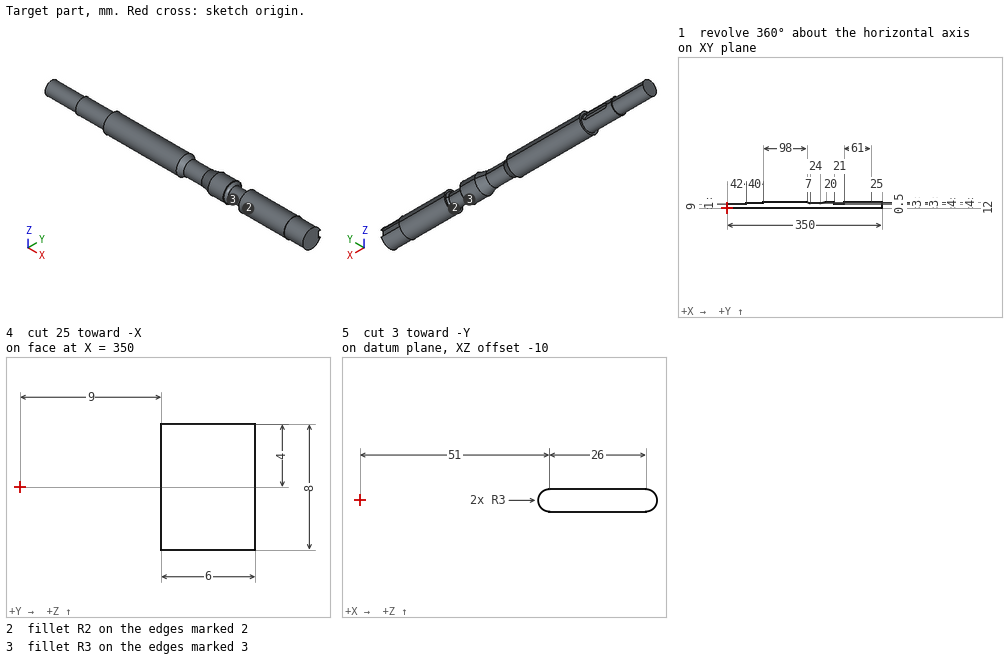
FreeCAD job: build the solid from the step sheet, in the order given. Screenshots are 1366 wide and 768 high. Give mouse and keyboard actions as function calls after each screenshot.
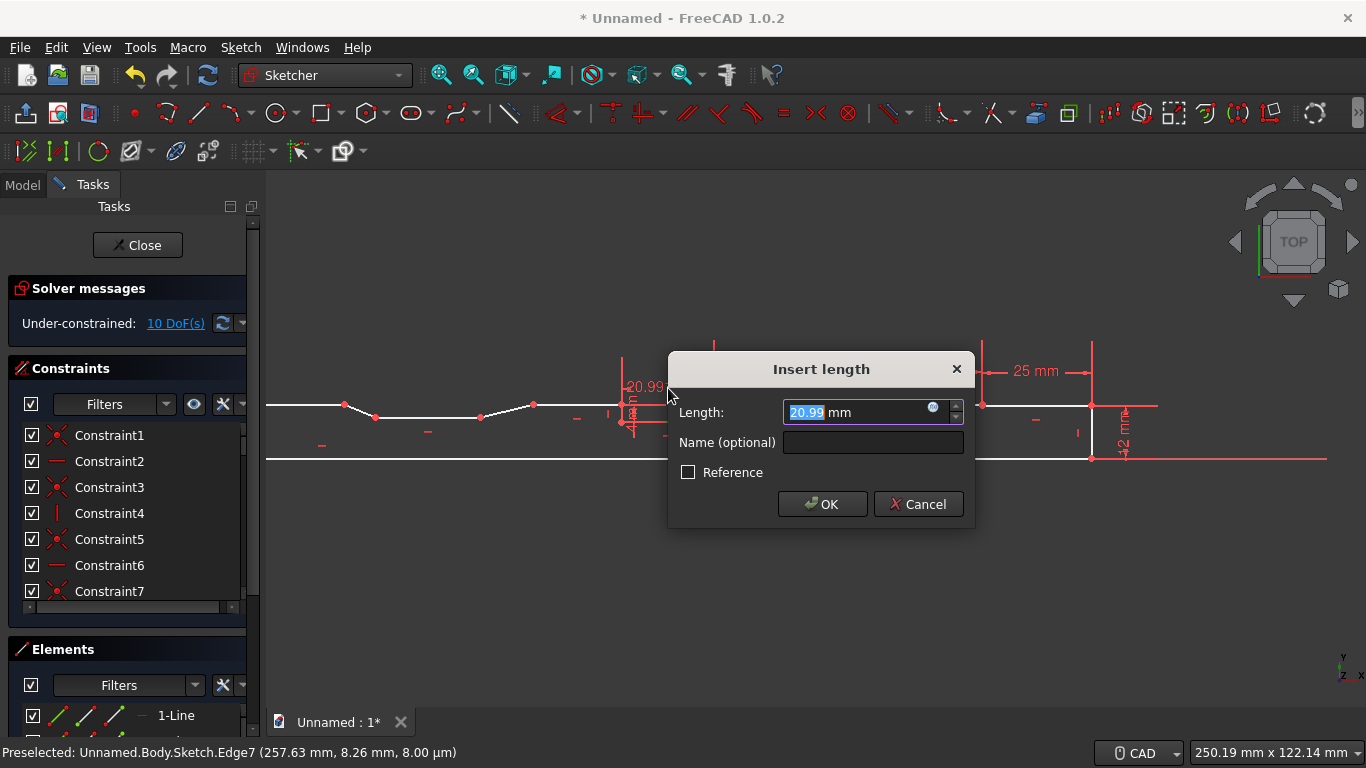
text(21)
key(Return)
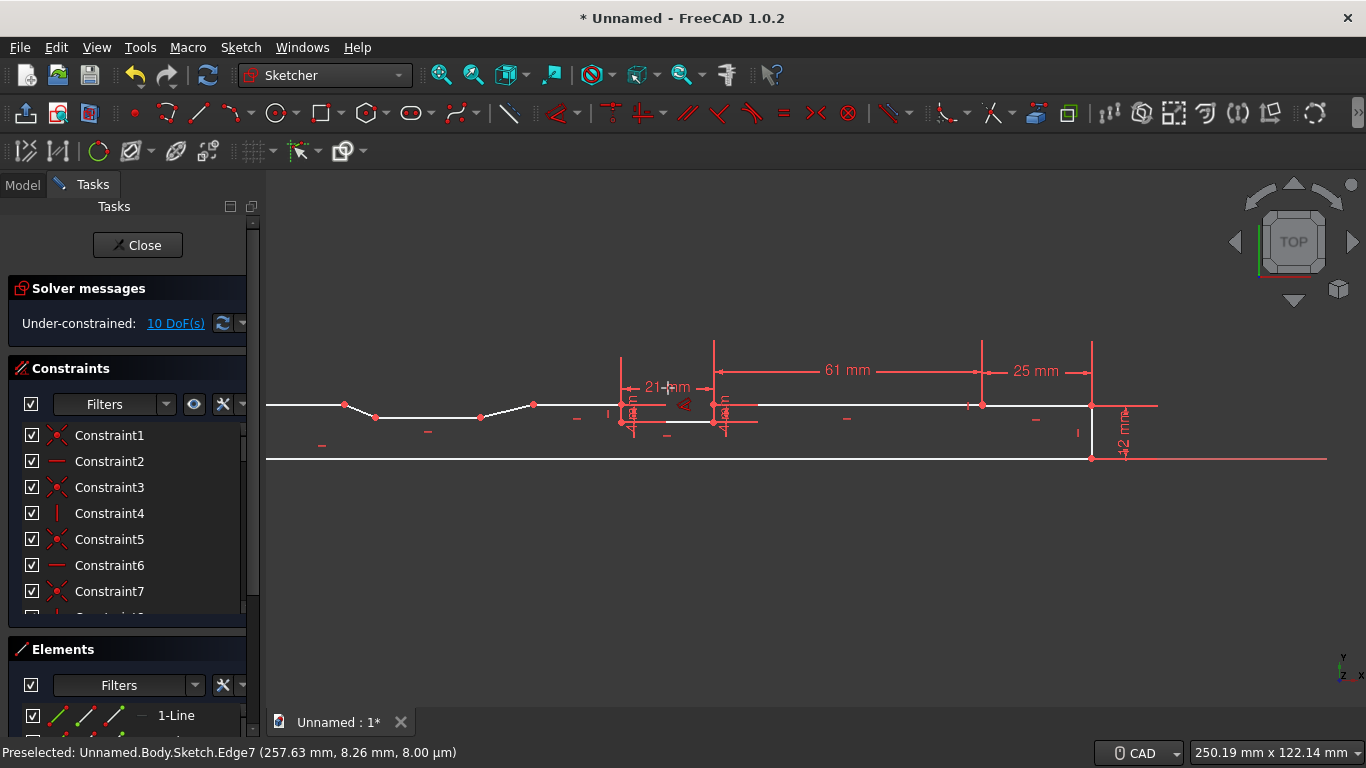
click(595, 405)
click(578, 371)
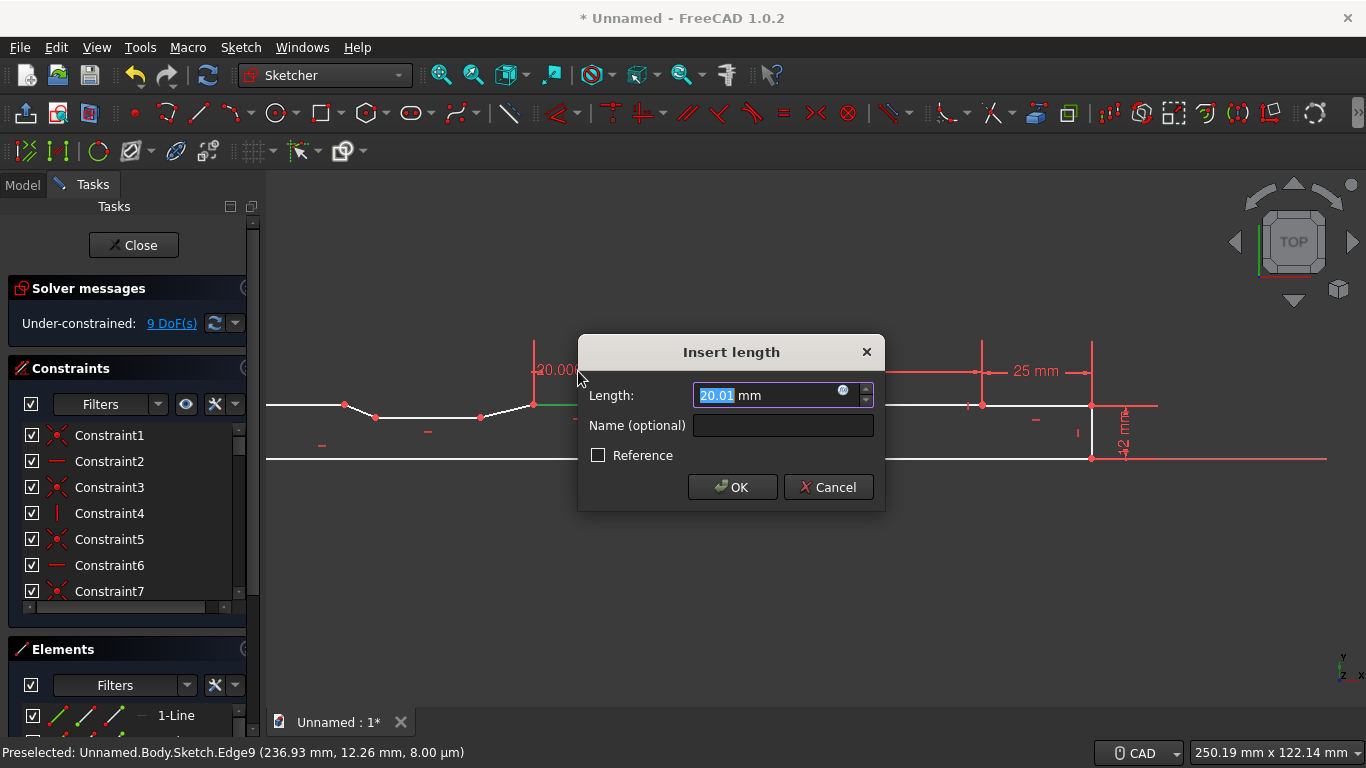
text(20)
key(Return)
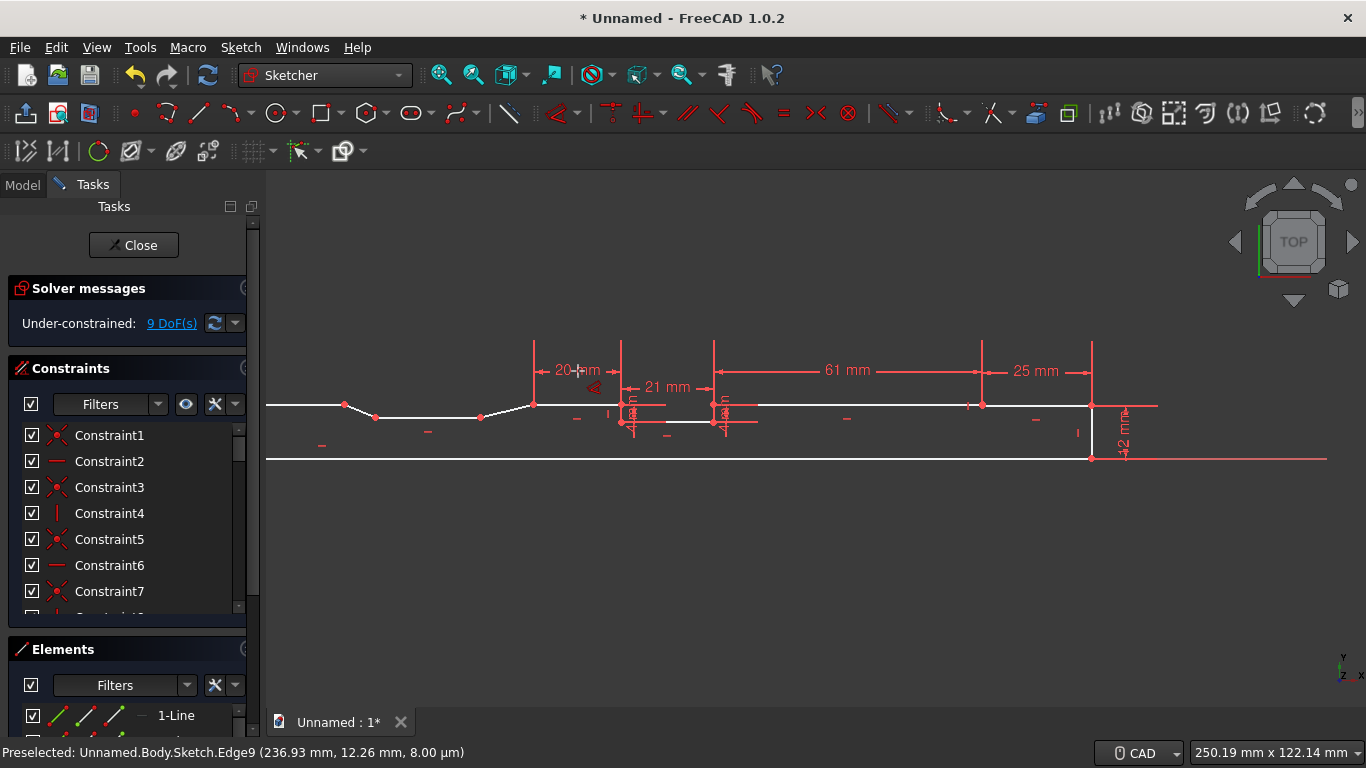
click(449, 418)
click(428, 384)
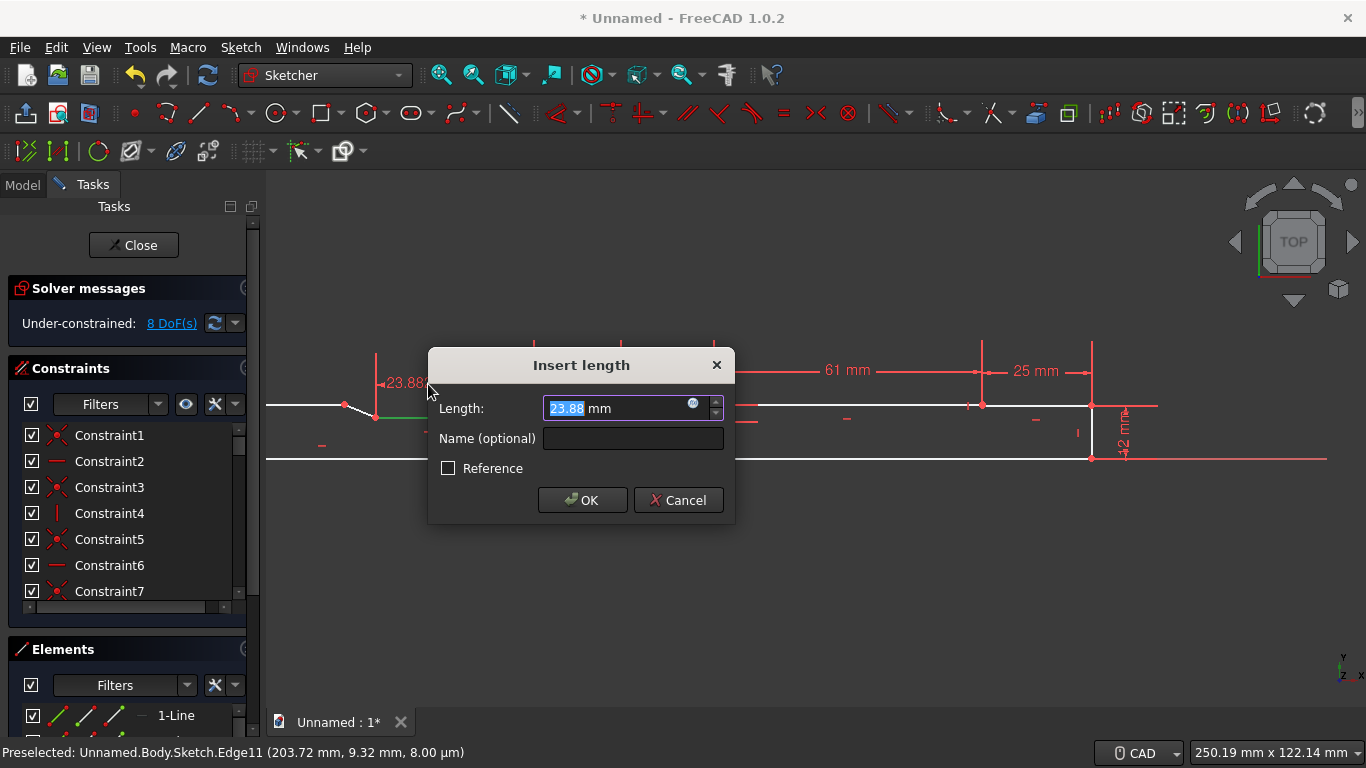
text(24)
key(Return)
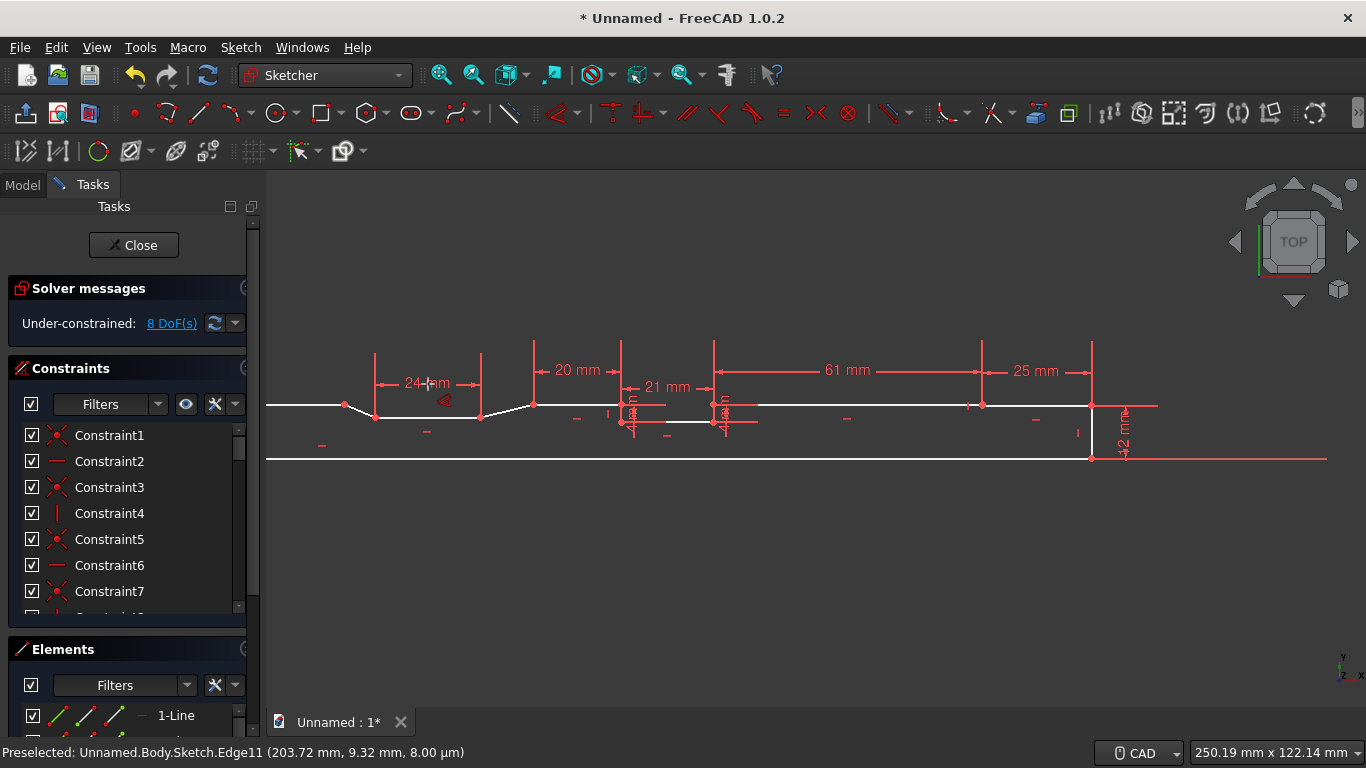
scroll(1094, 445, down, 4)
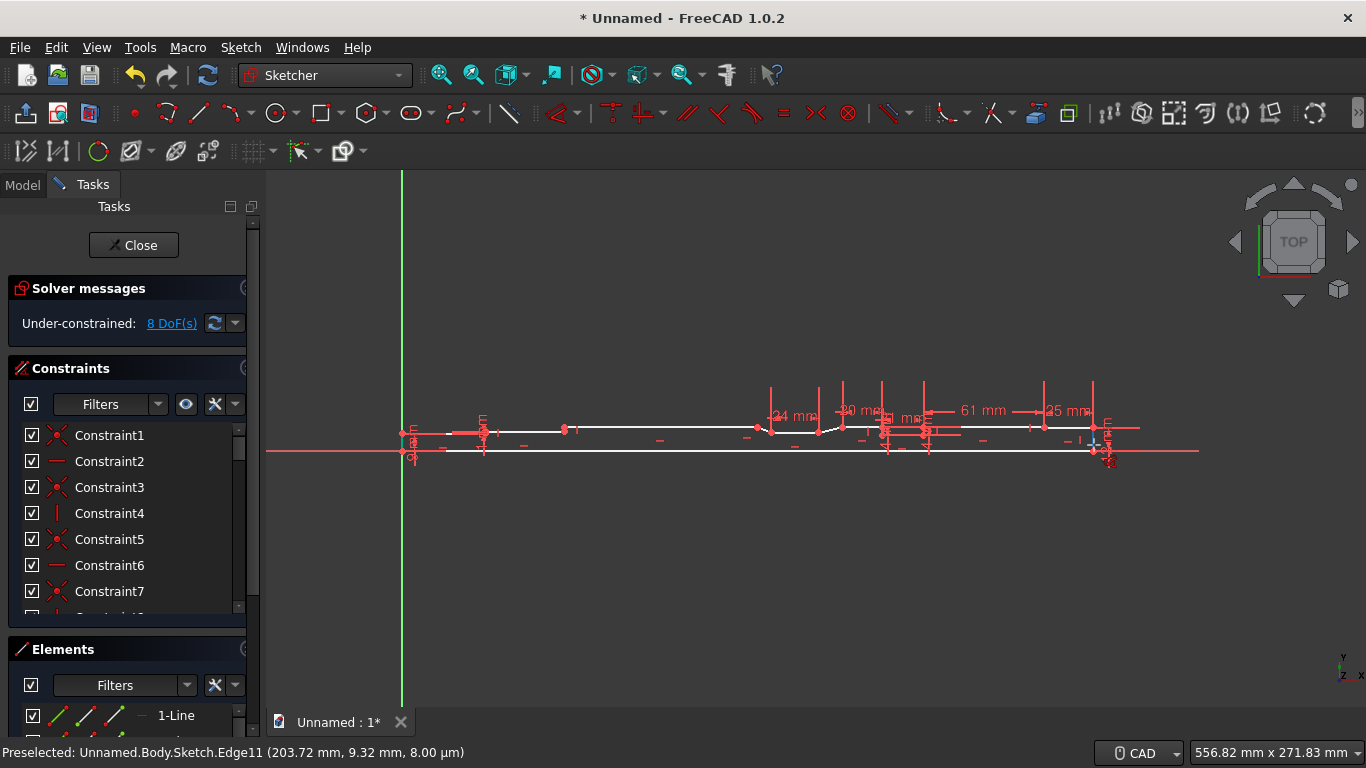
click(700, 427)
click(661, 393)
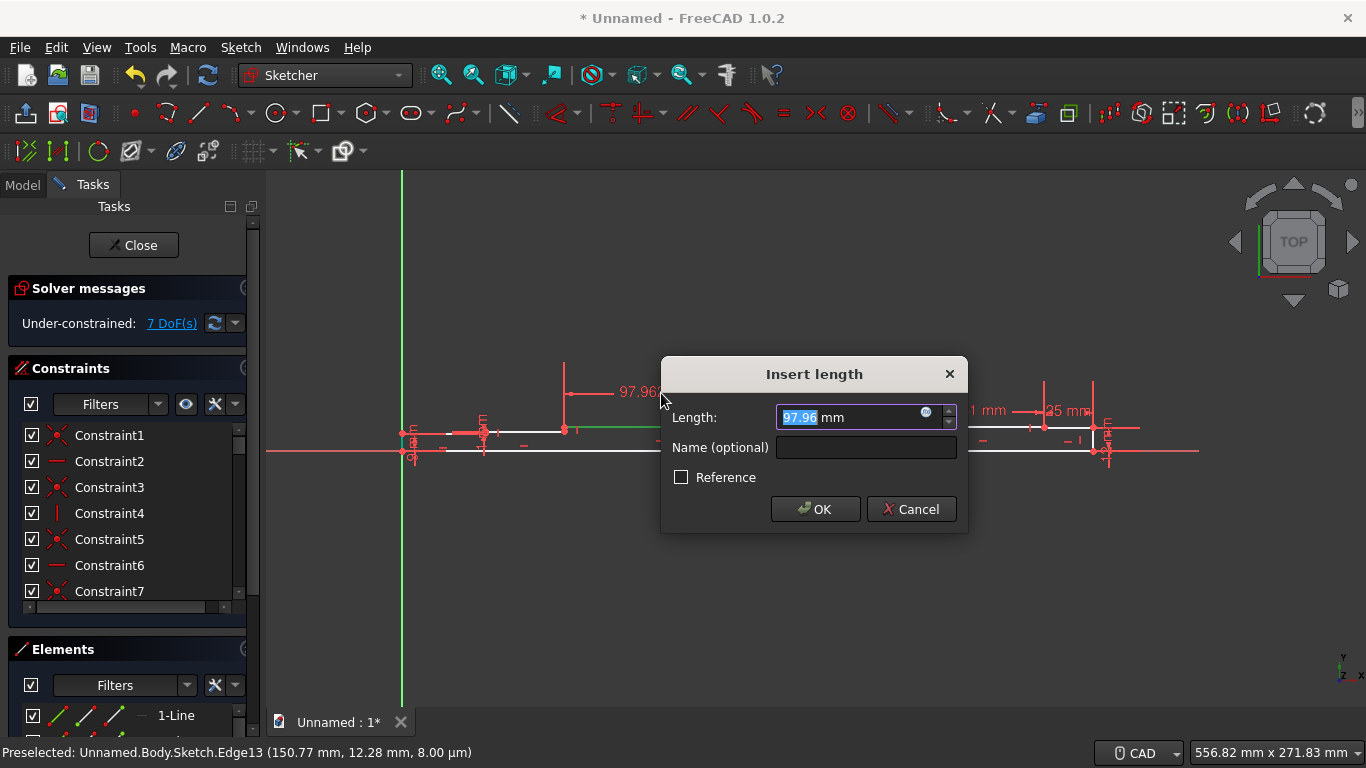
text(98)
key(Return)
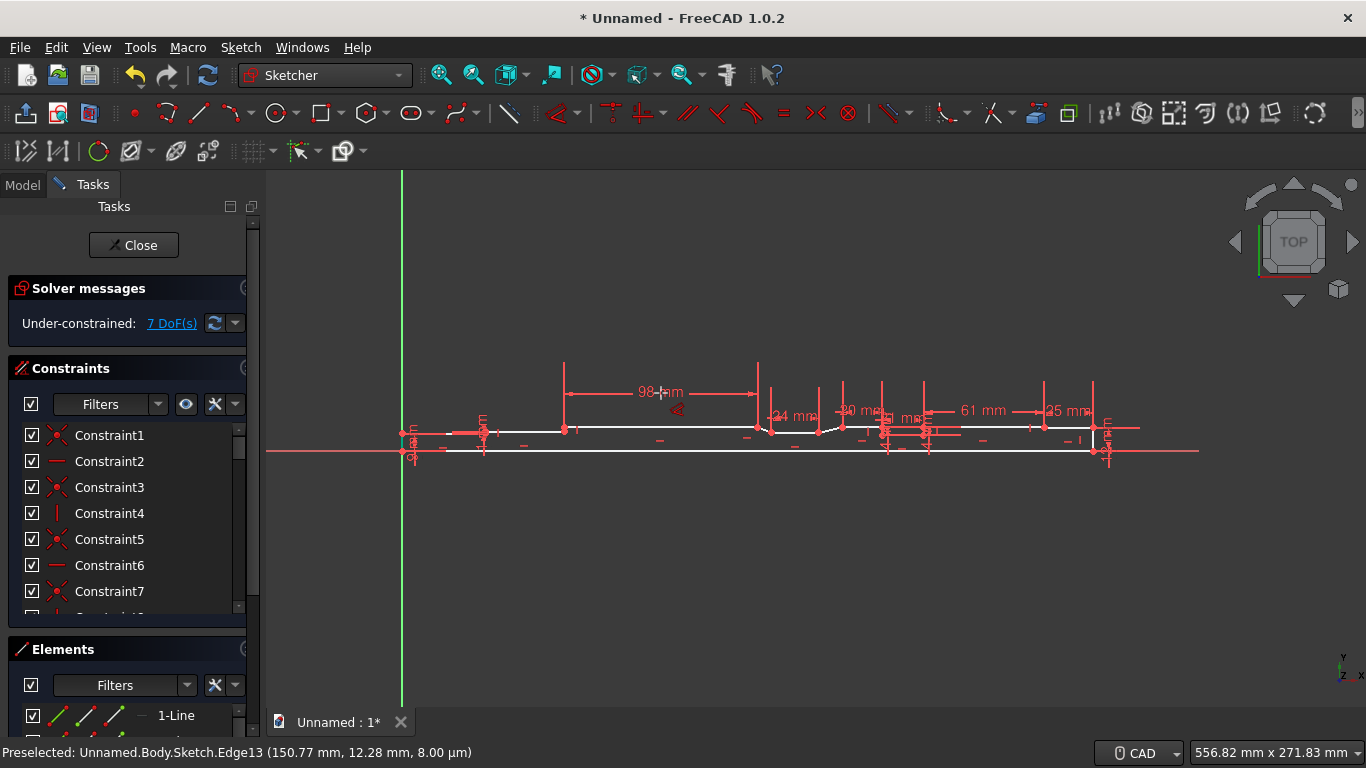
click(540, 432)
click(525, 398)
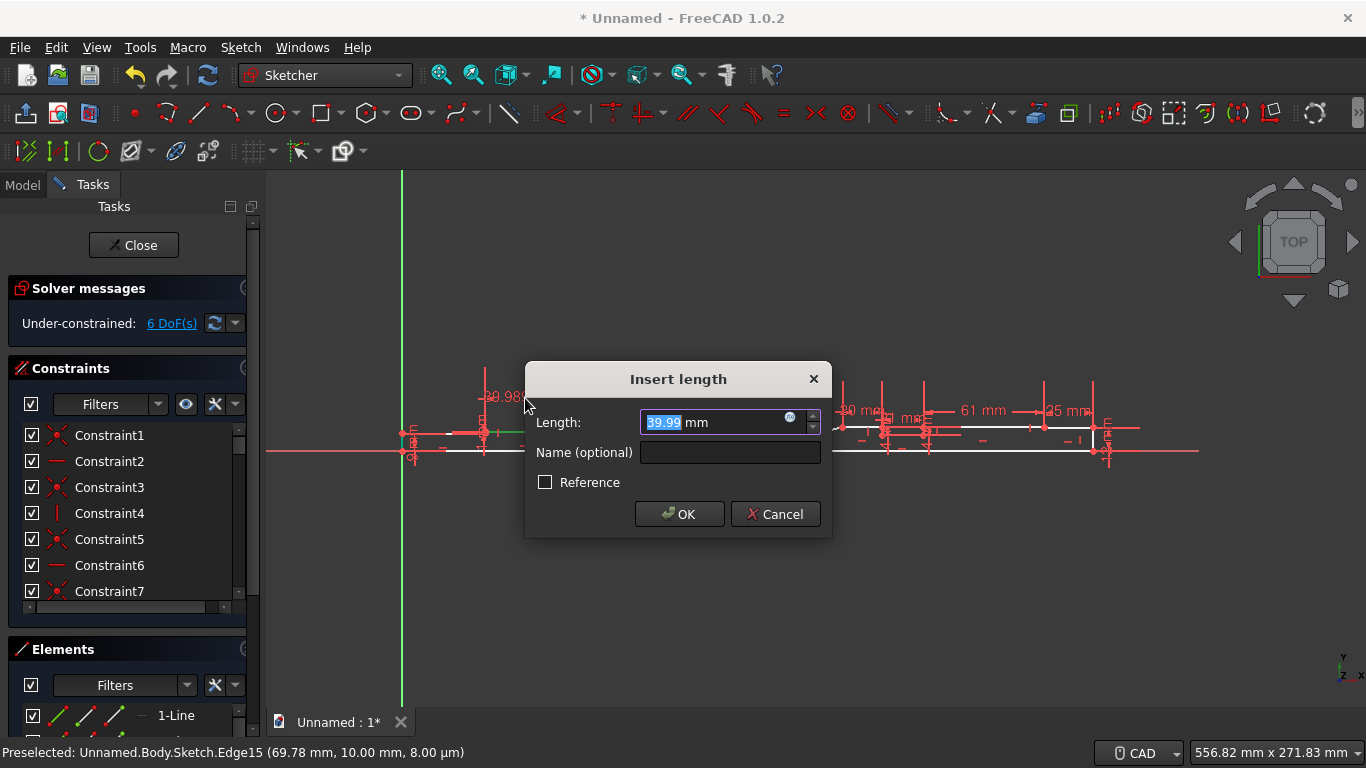
text(40)
key(Return)